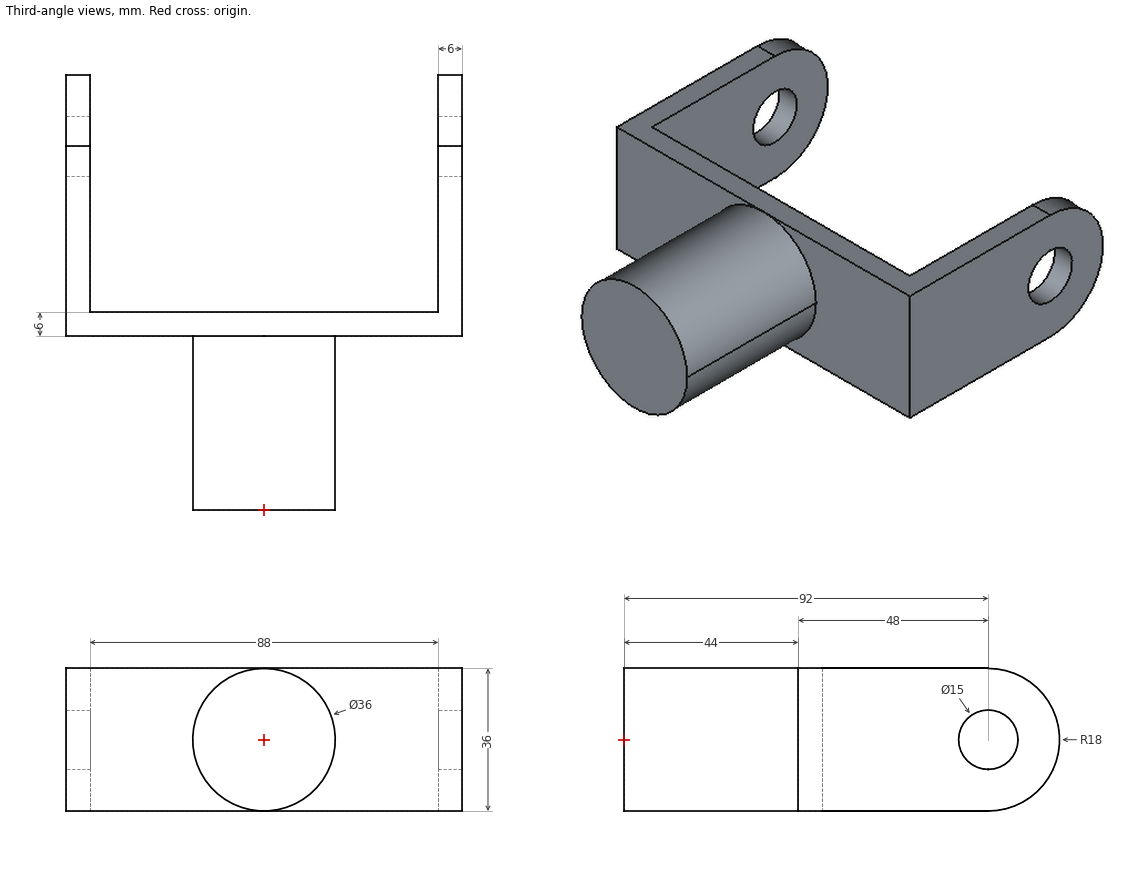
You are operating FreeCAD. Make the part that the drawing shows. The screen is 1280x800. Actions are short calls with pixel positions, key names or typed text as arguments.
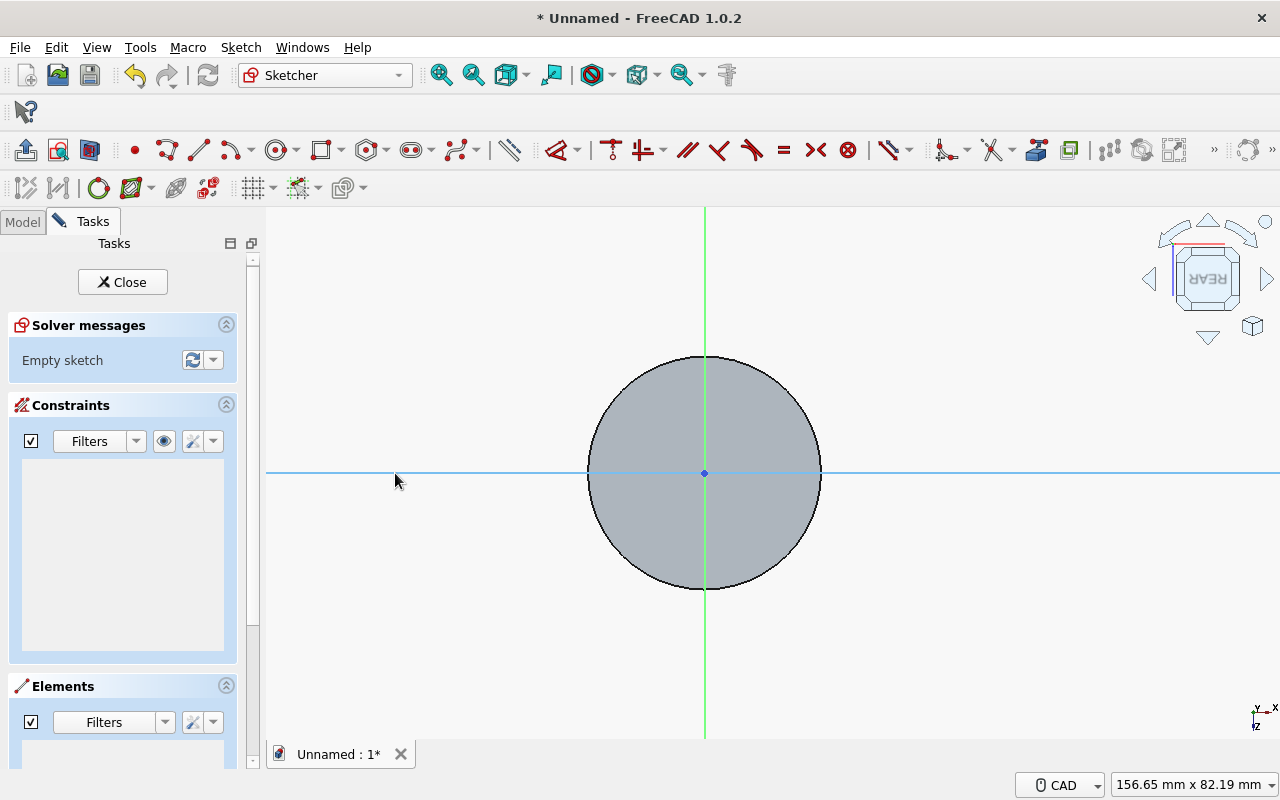
key(g)
key(v)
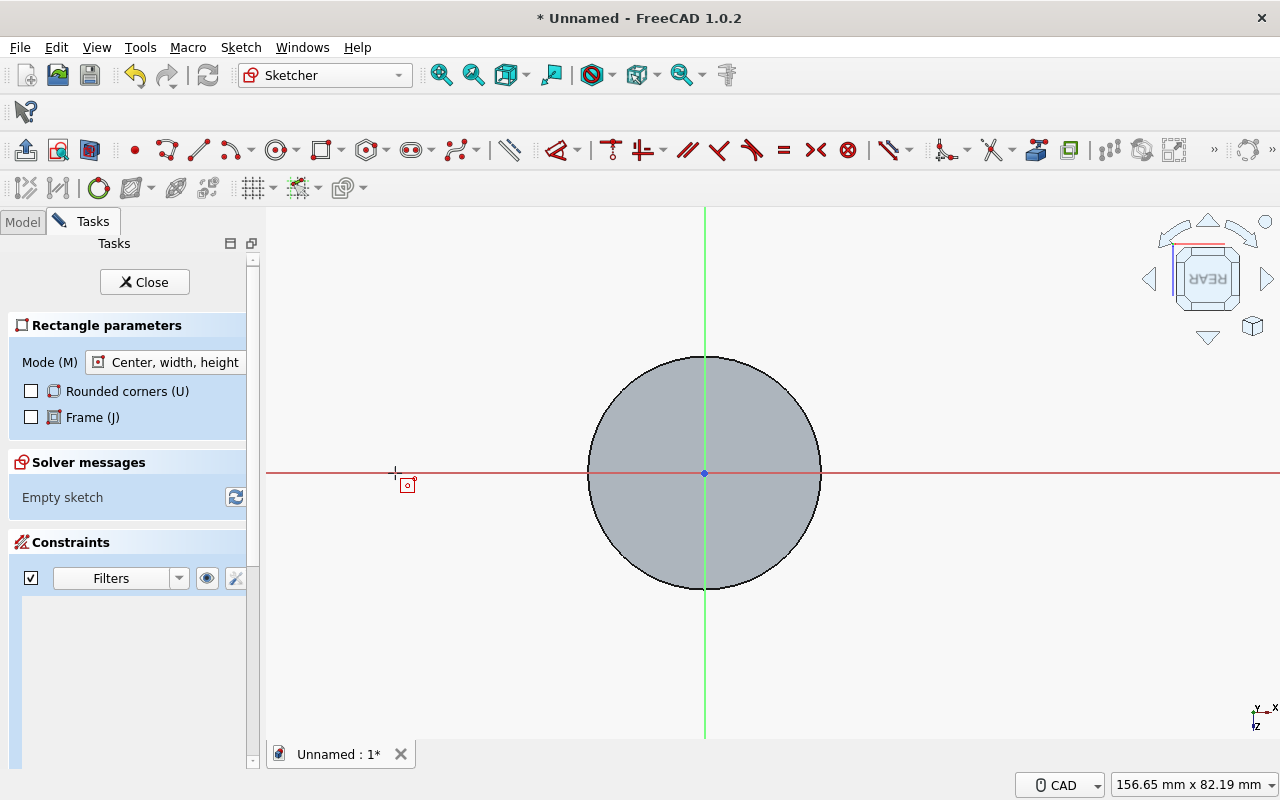
click(705, 473)
click(989, 357)
key(Escape)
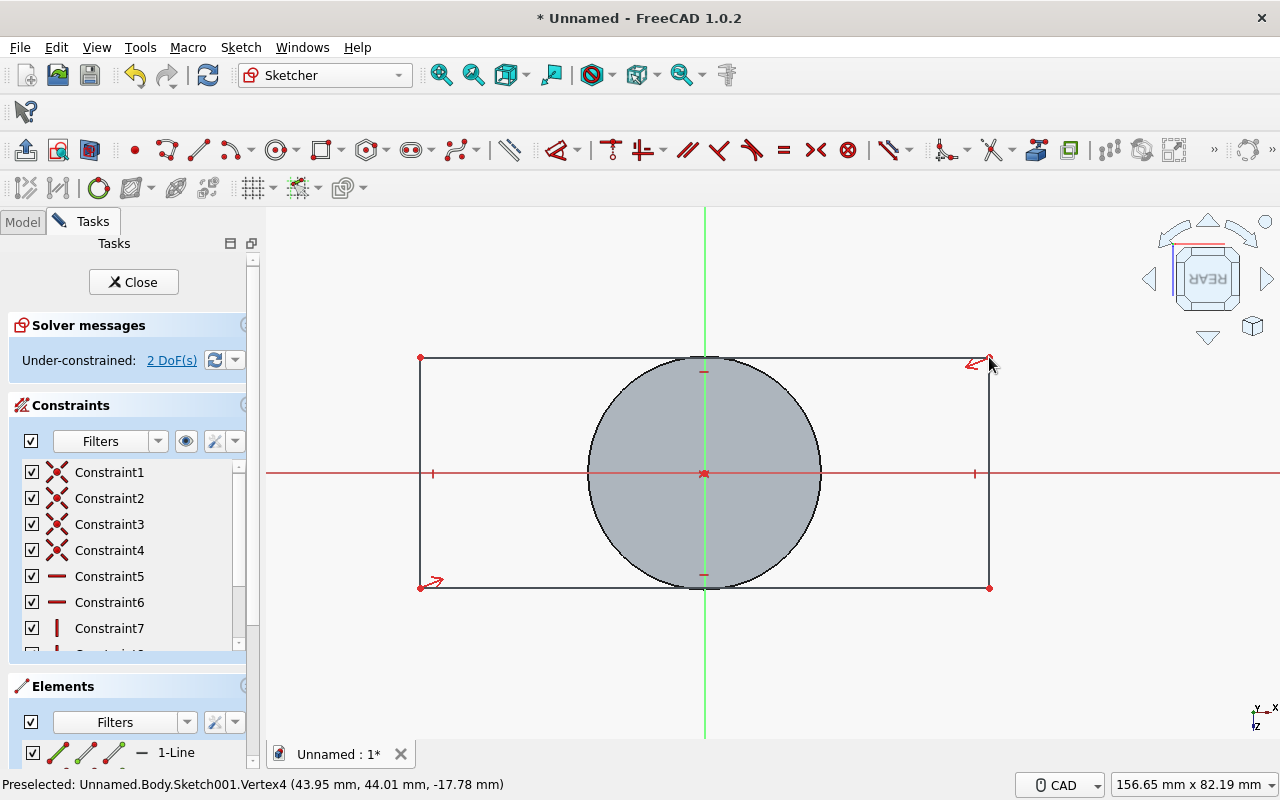
click(591, 588)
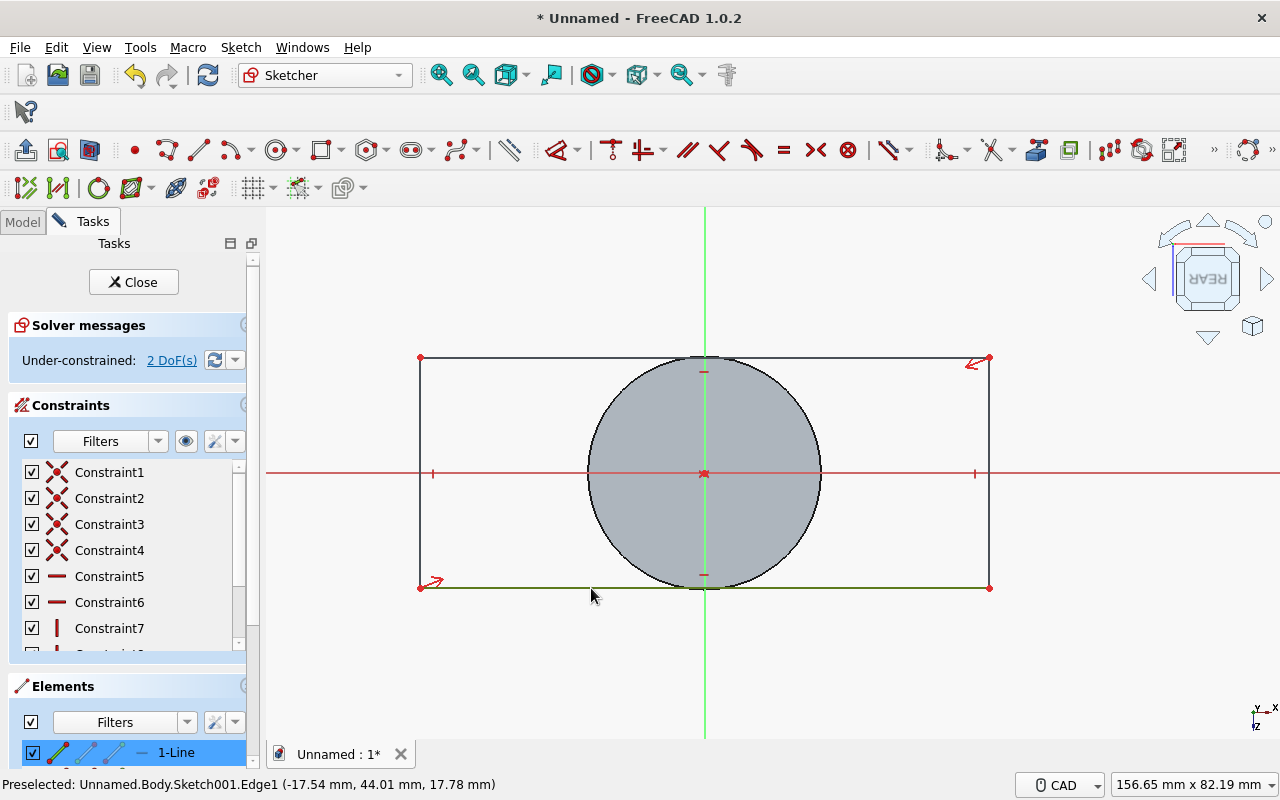
key(l)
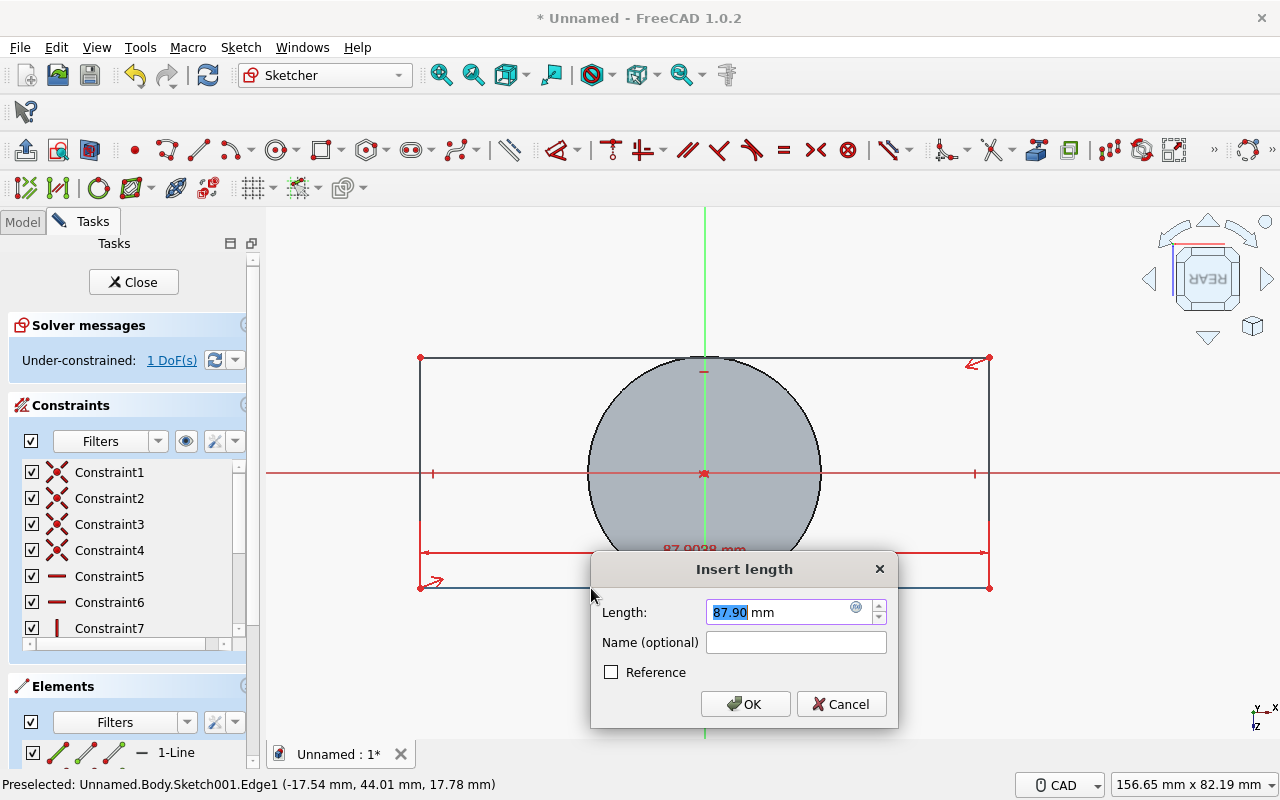
text(88)
key(Return)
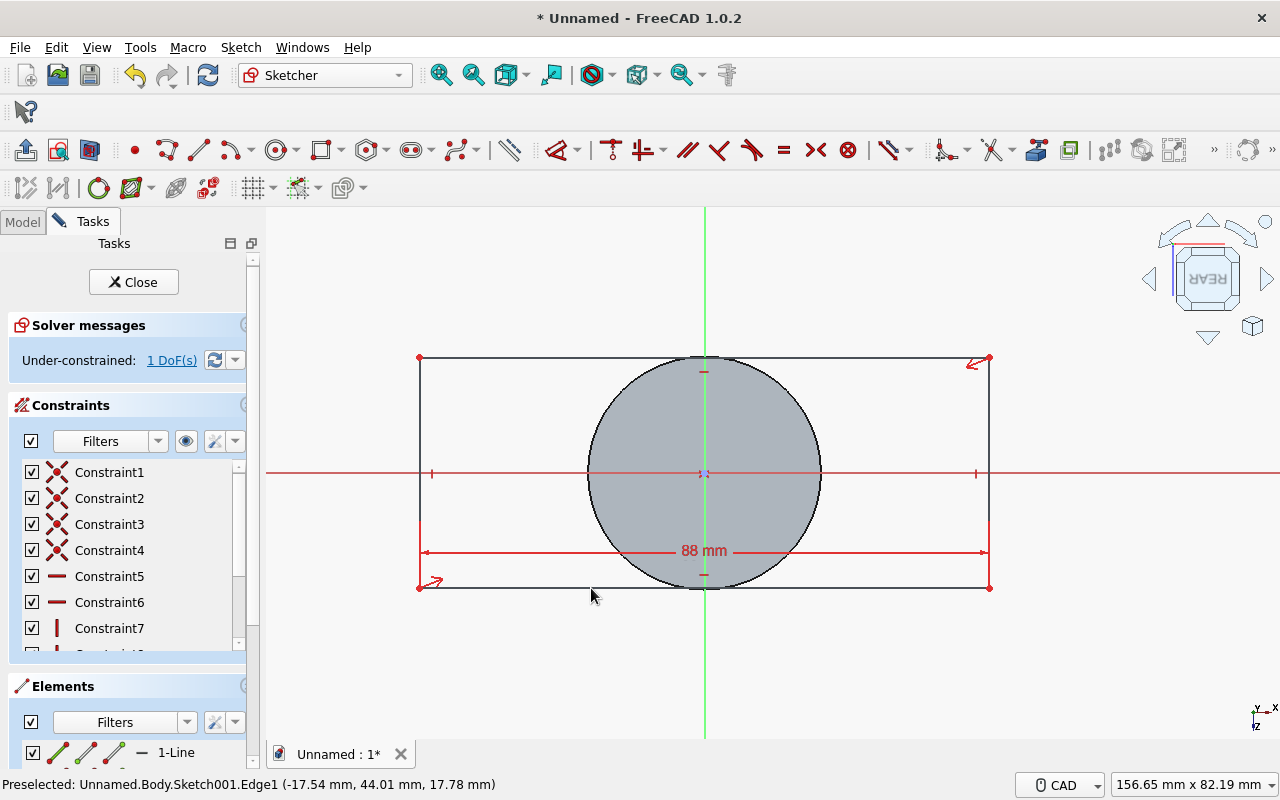
click(989, 519)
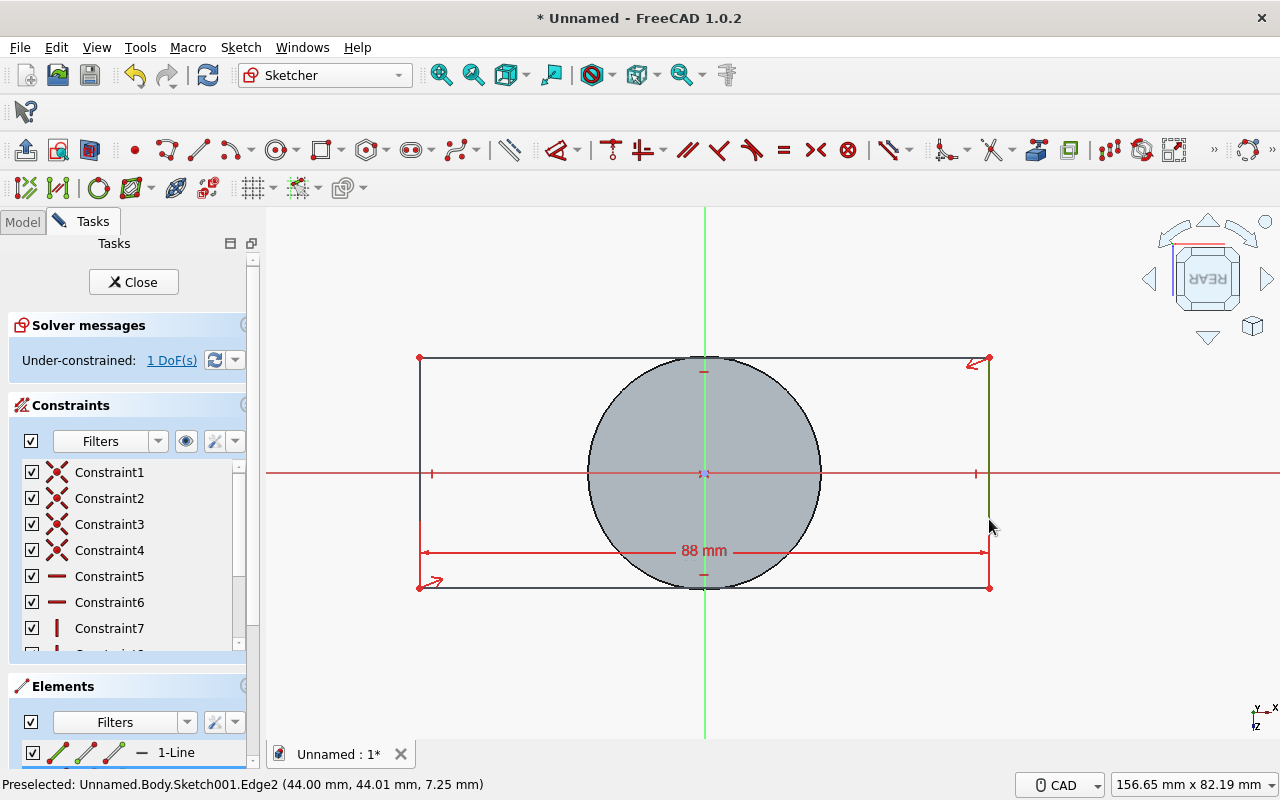
key(i)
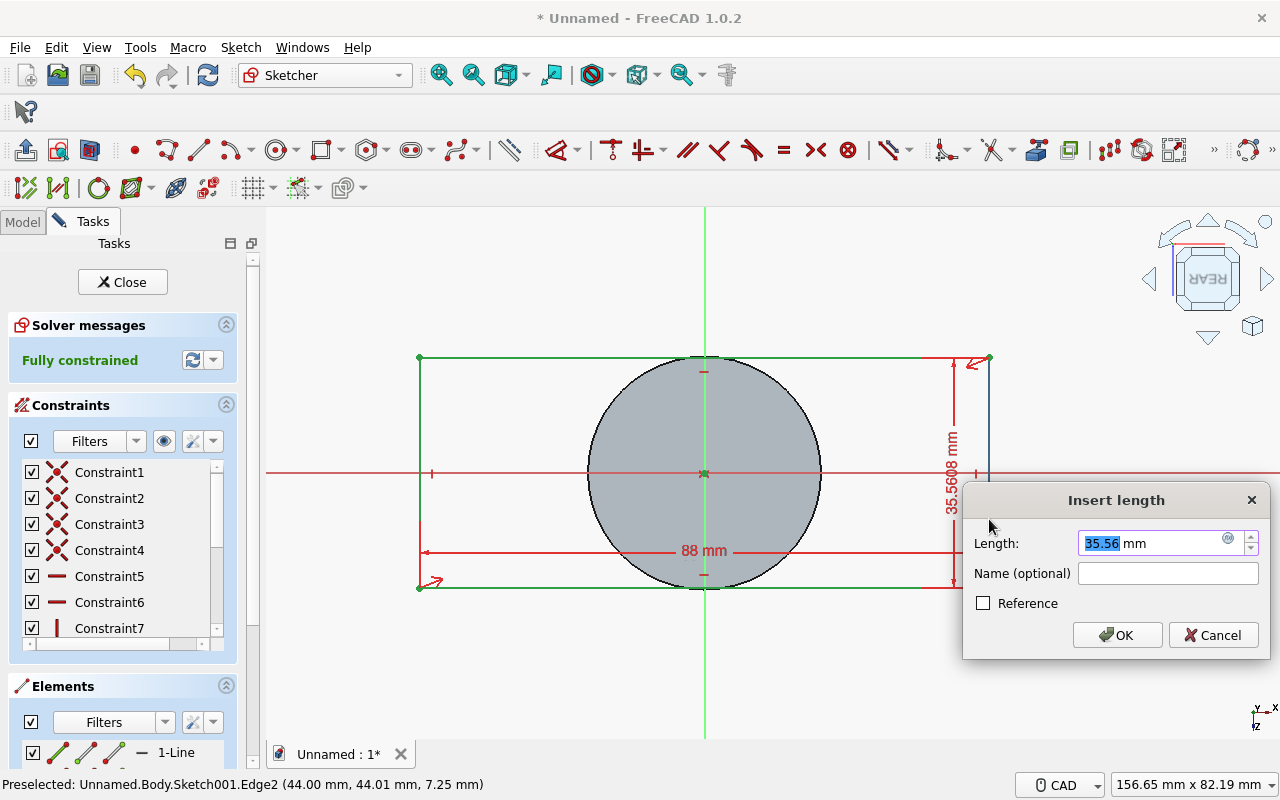
text(36)
key(Return)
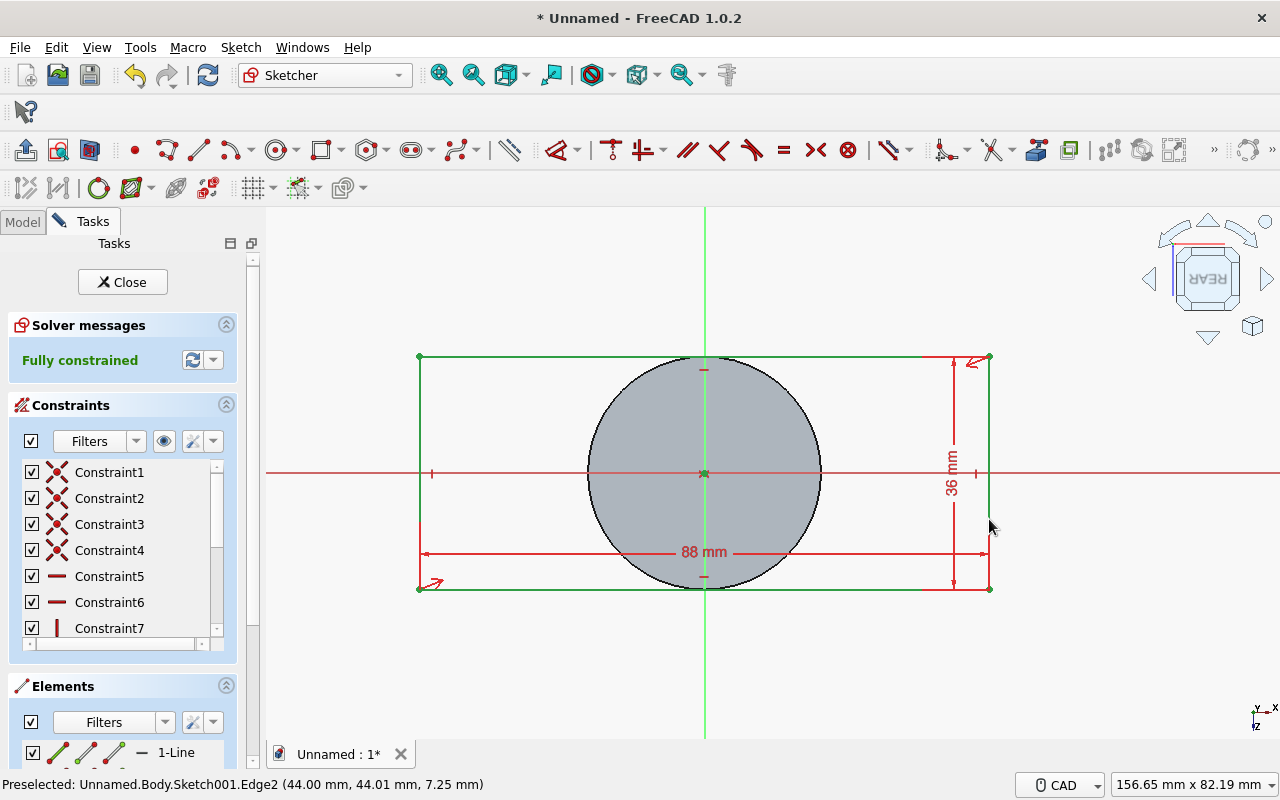
click(123, 282)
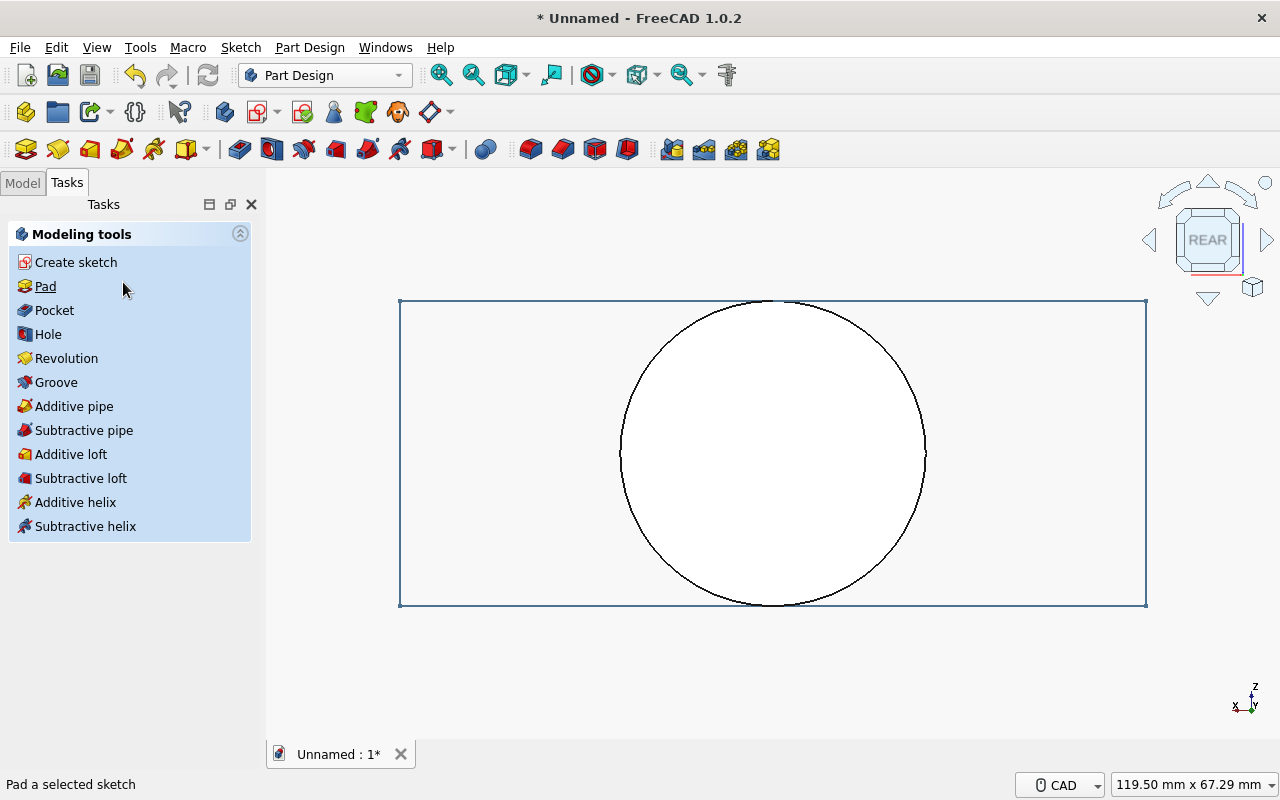
click(26, 150)